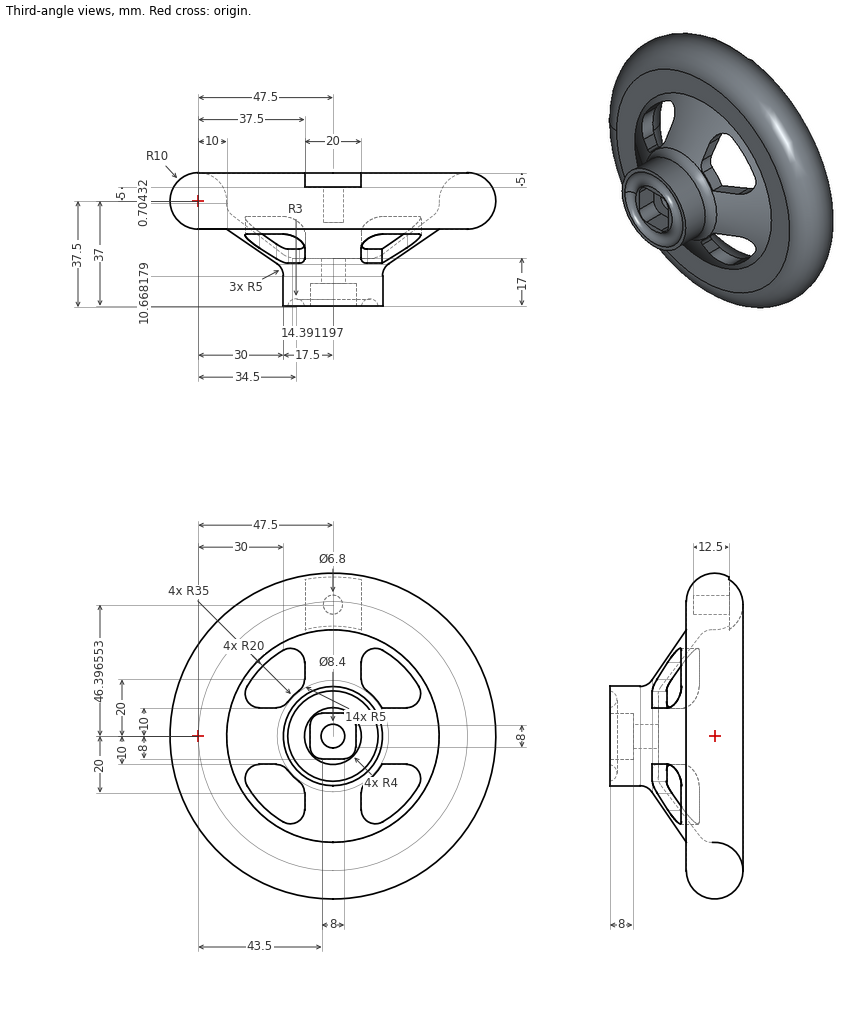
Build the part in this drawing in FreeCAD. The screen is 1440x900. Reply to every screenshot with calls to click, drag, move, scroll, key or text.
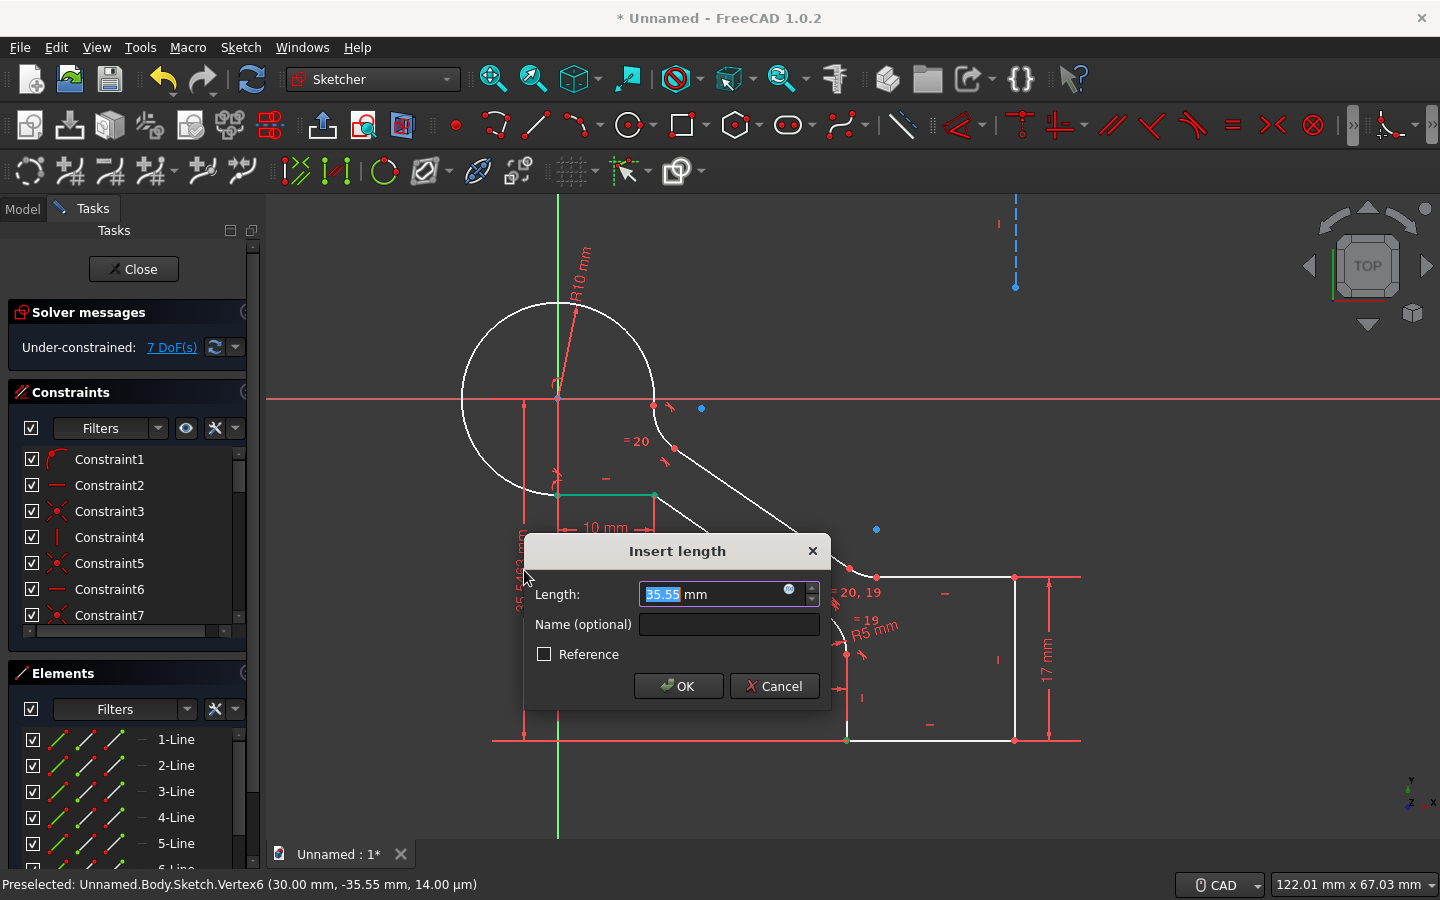
text(37)
key(Return)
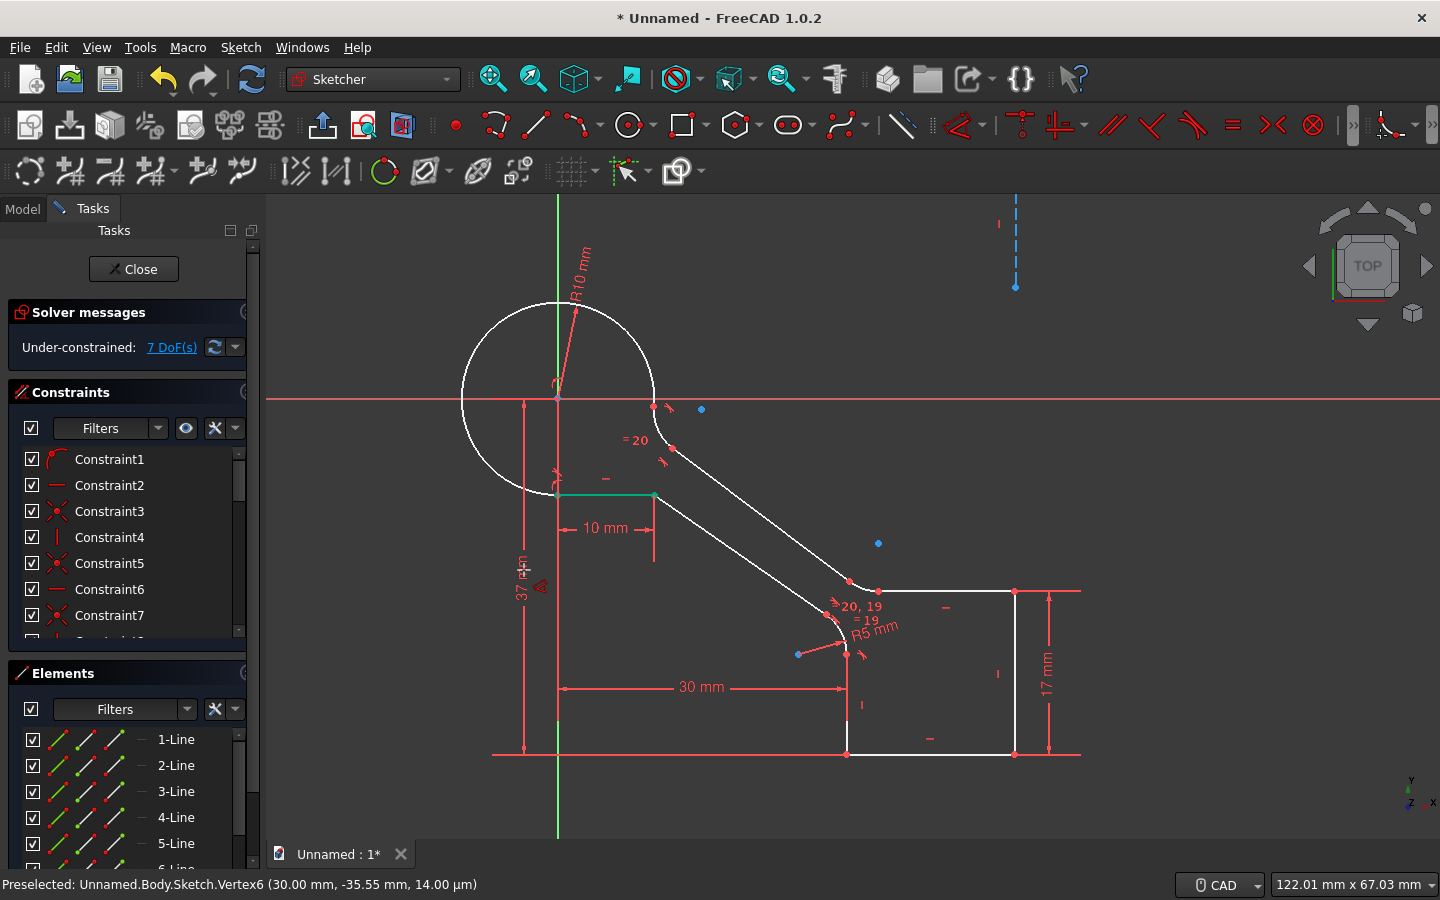
click(897, 755)
click(931, 789)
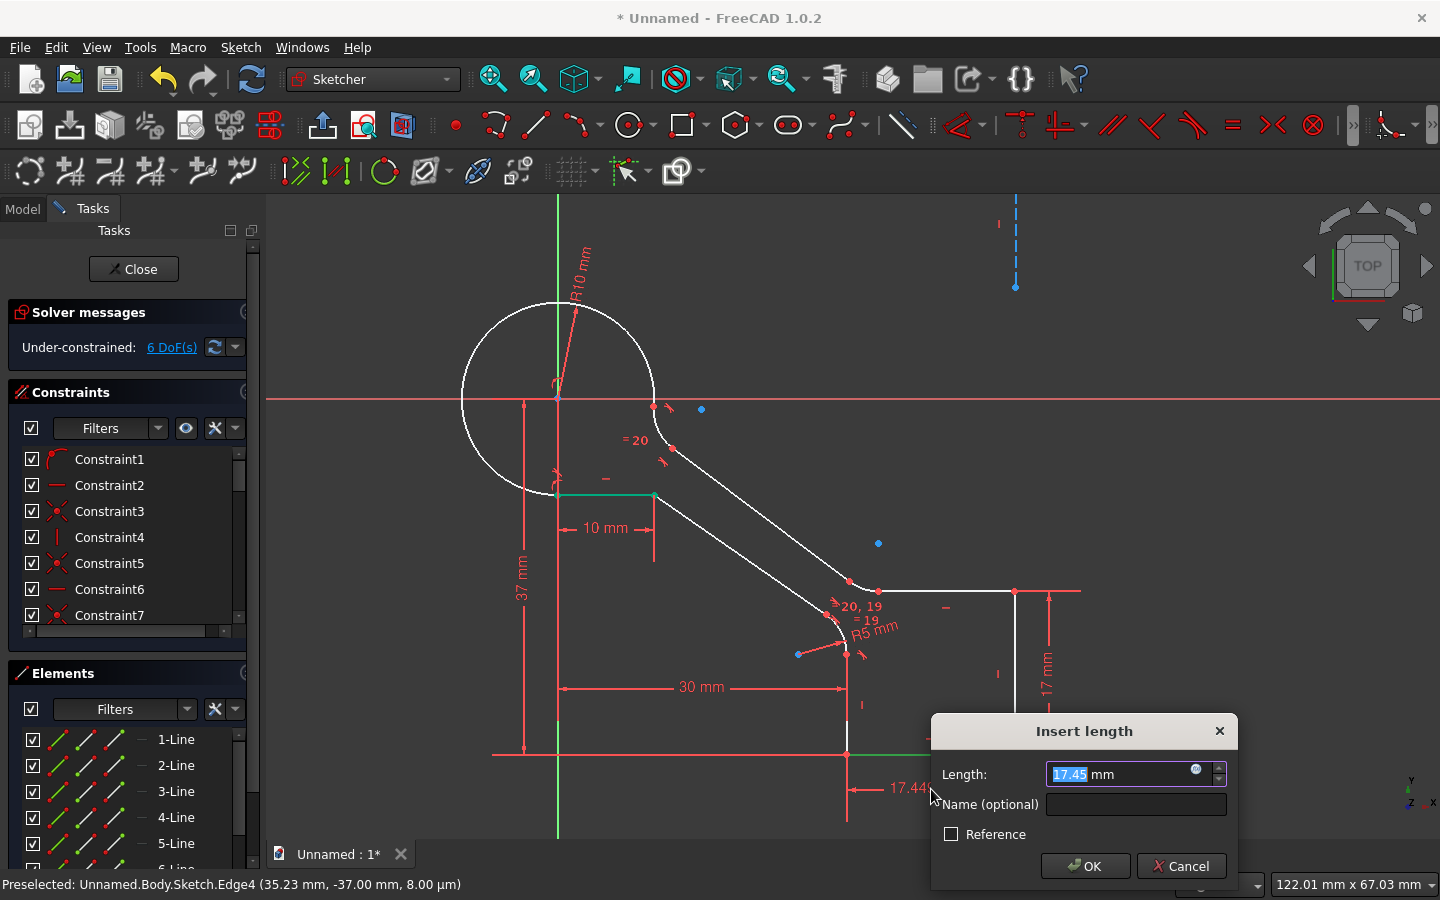
text(17.5)
key(Return)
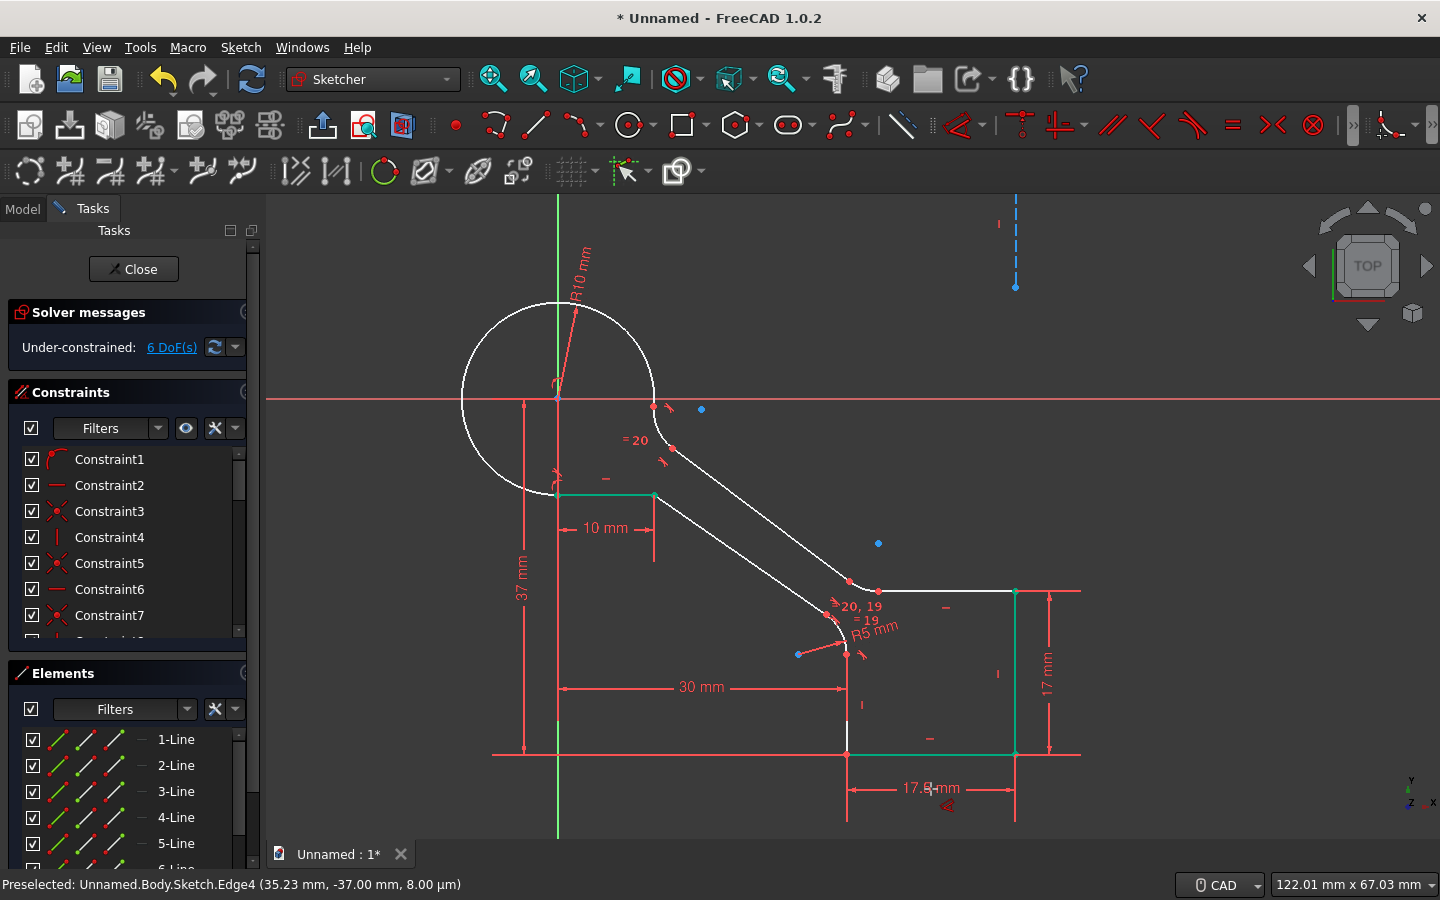
click(1016, 287)
click(787, 253)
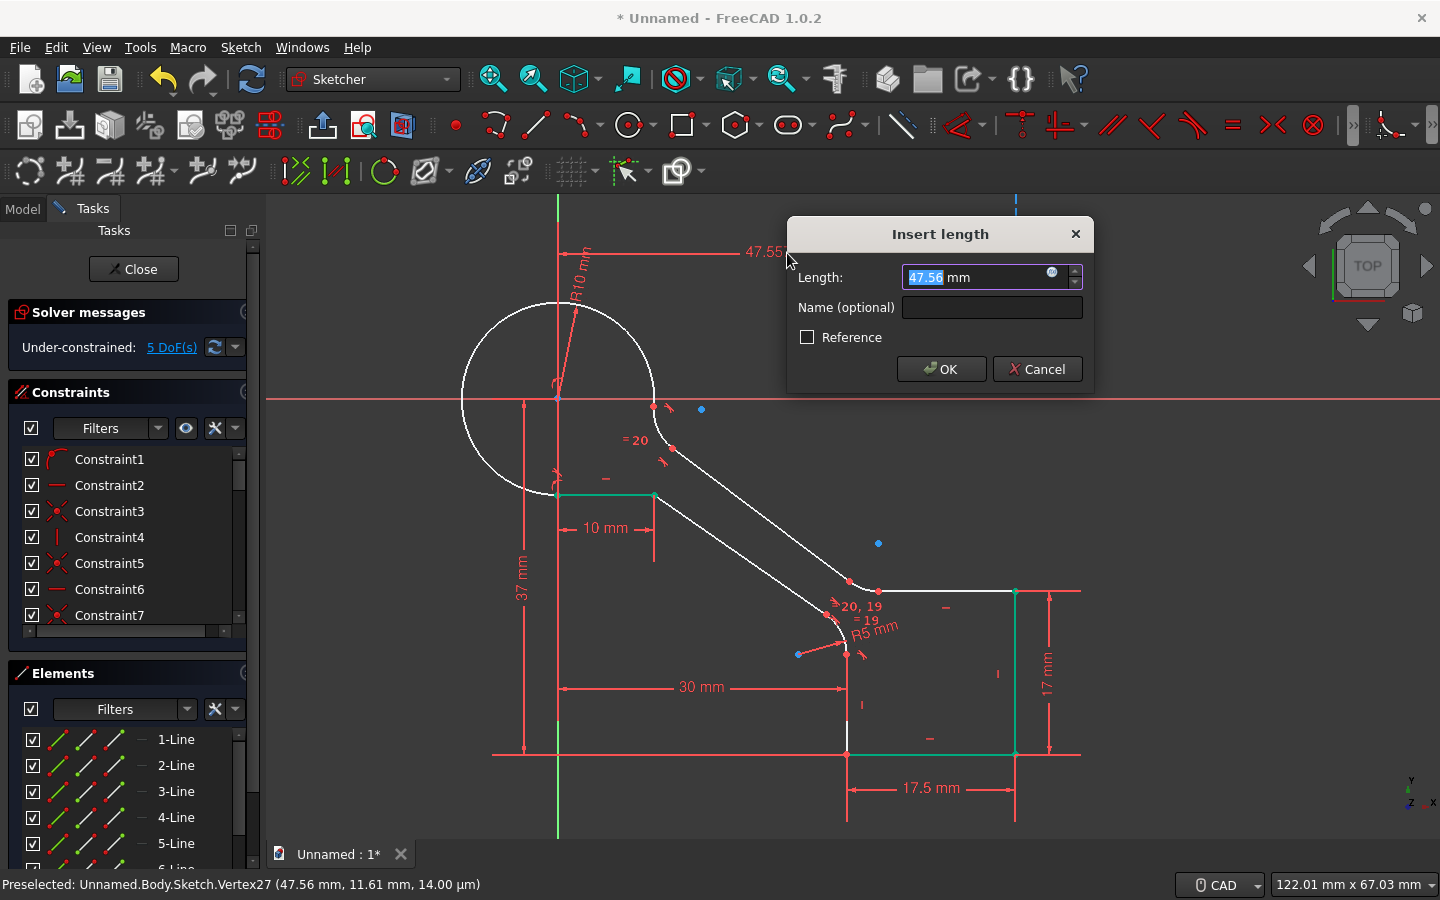
text(47.5)
key(Return)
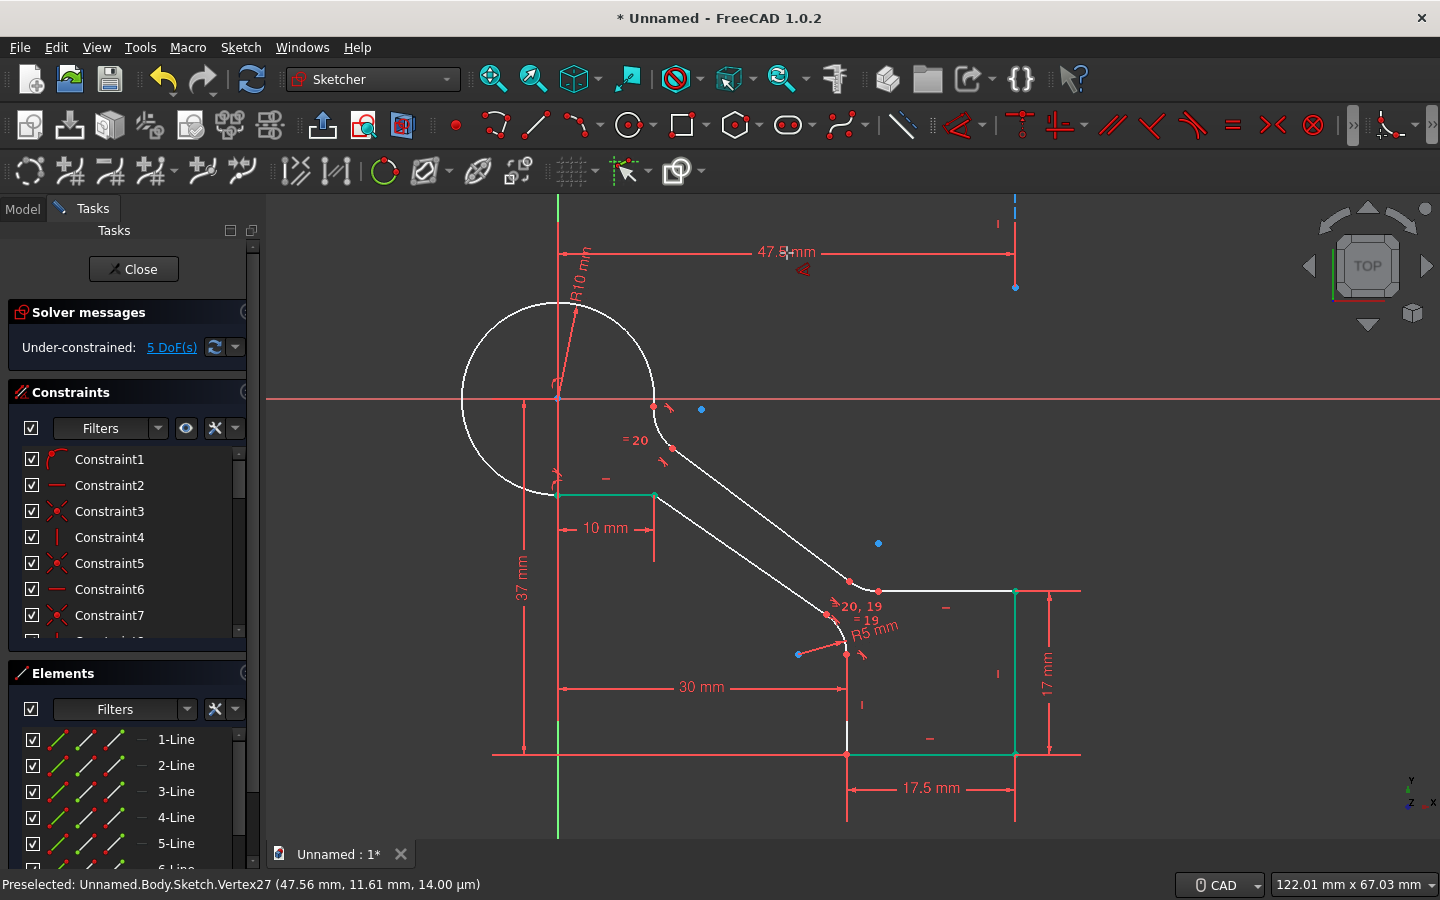
scroll(654, 406, up, 9)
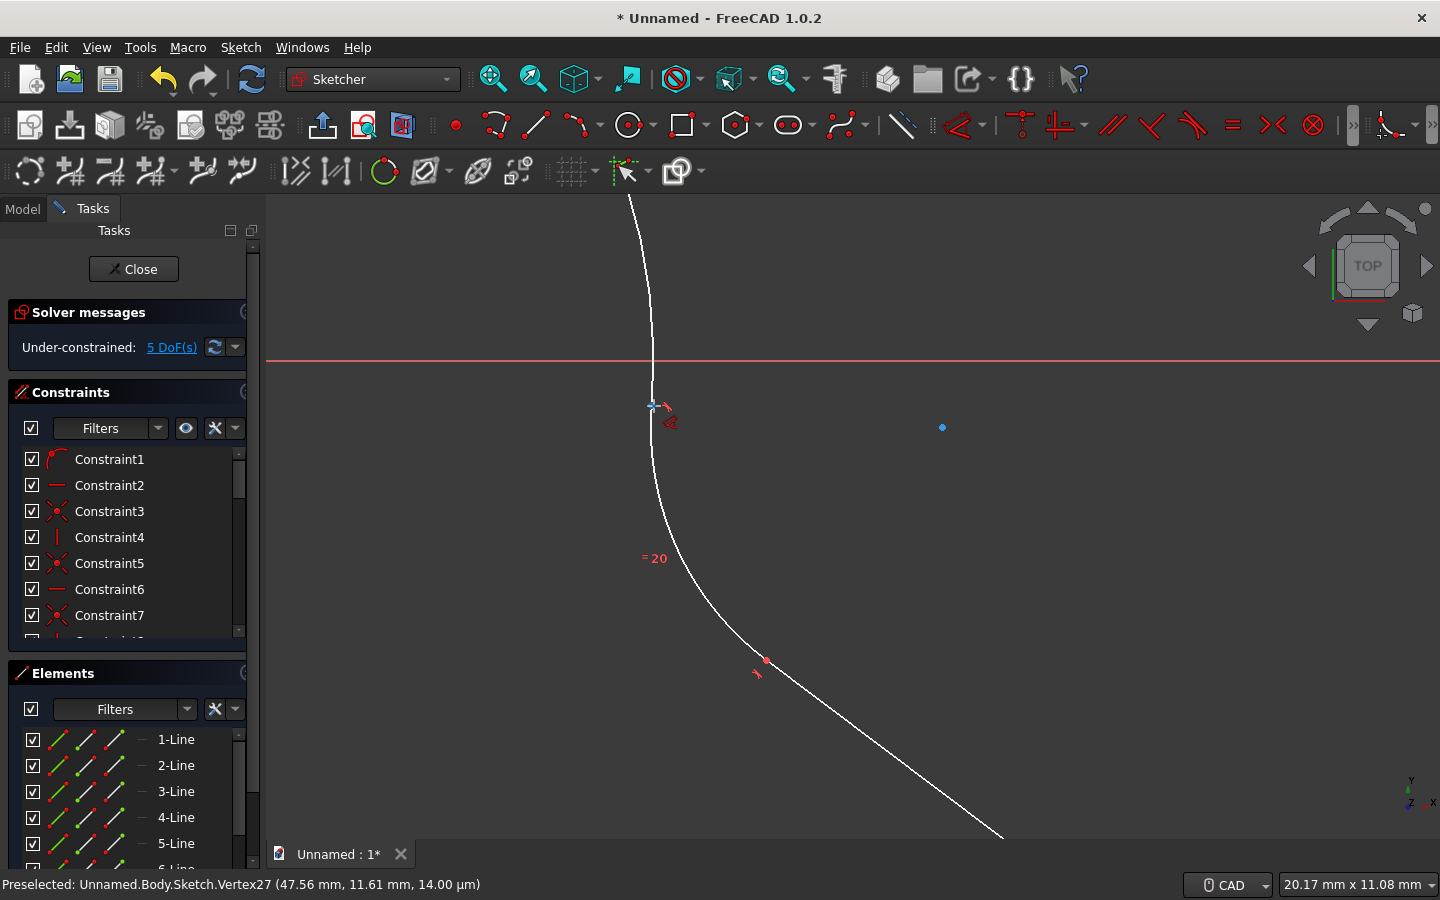
click(652, 406)
click(686, 384)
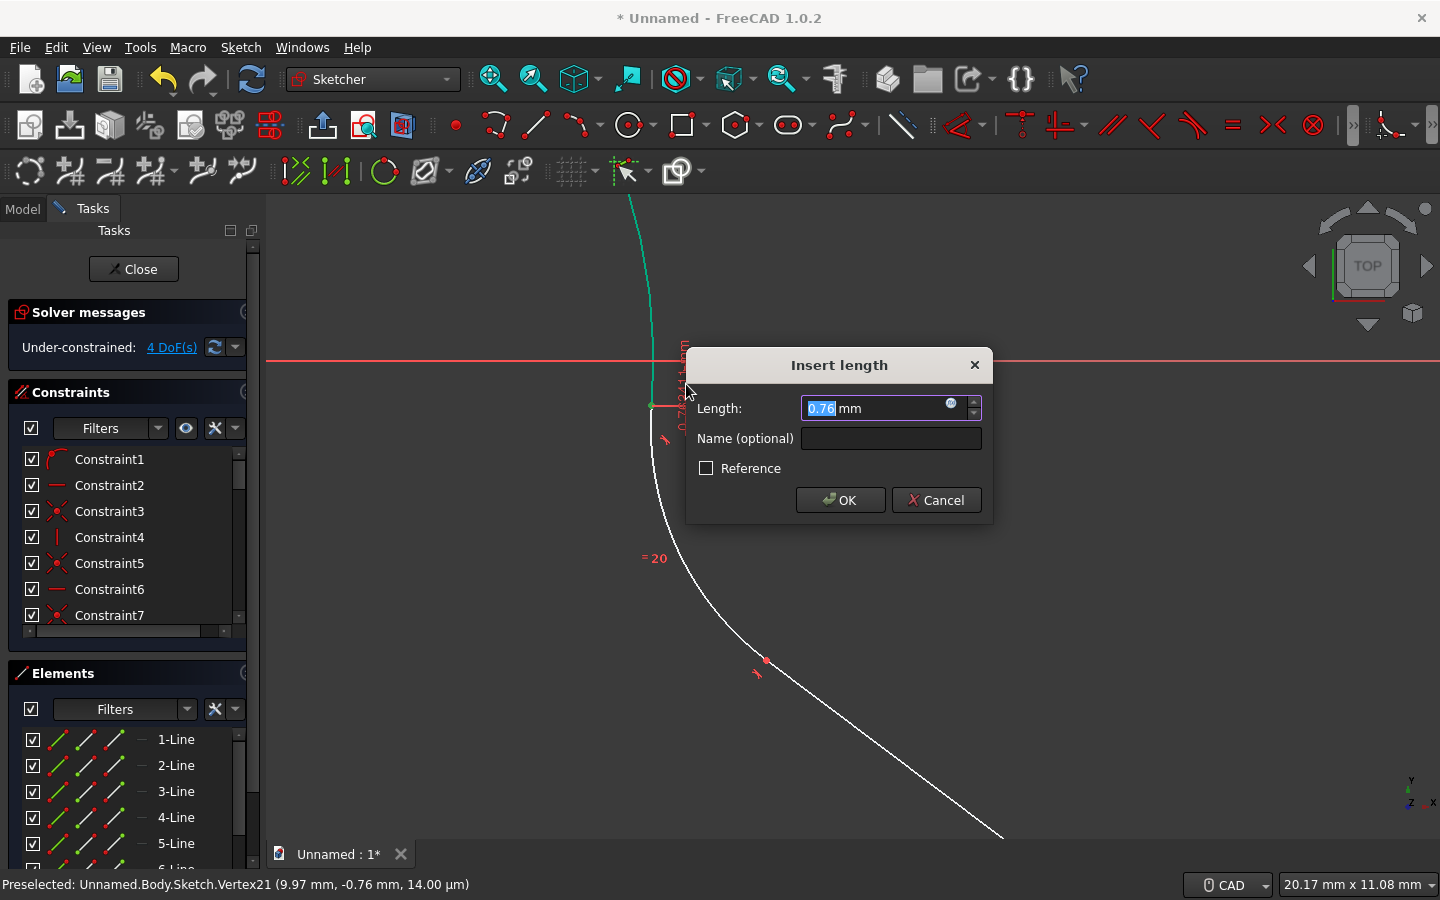
text(0.70432)
key(Return)